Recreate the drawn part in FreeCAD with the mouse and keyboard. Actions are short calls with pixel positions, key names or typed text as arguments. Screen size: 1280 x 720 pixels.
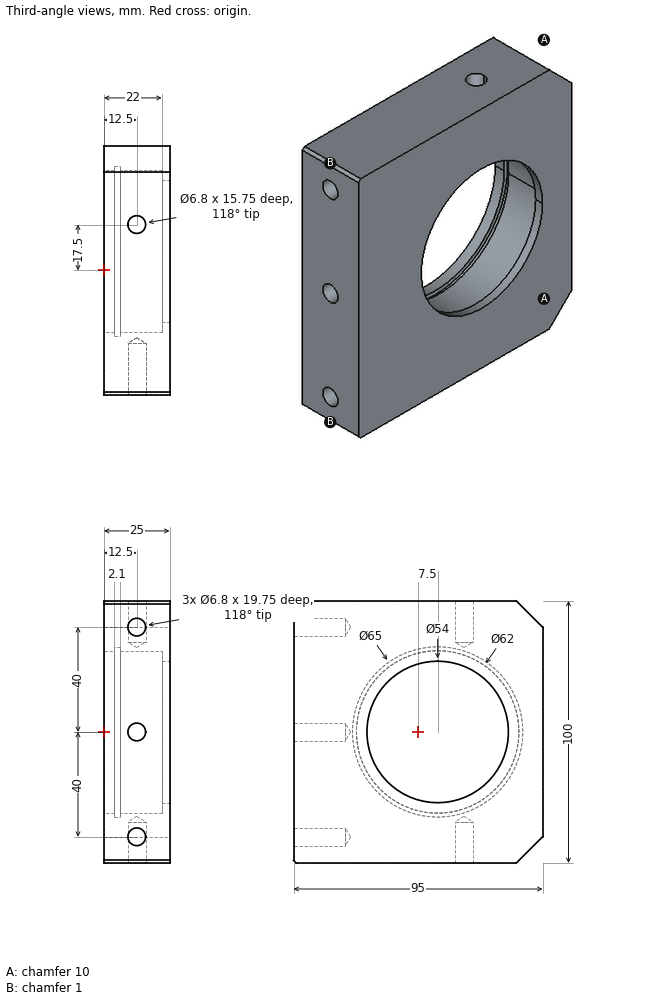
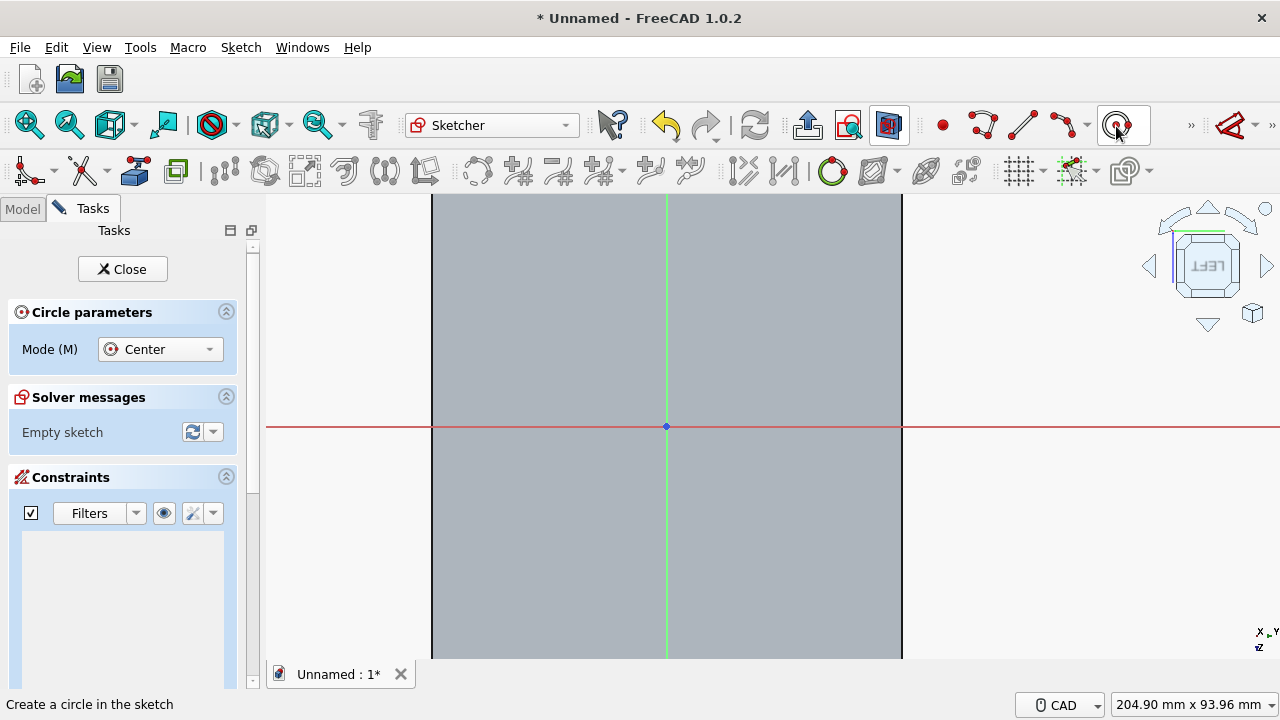
click(704, 426)
click(812, 318)
key(Escape)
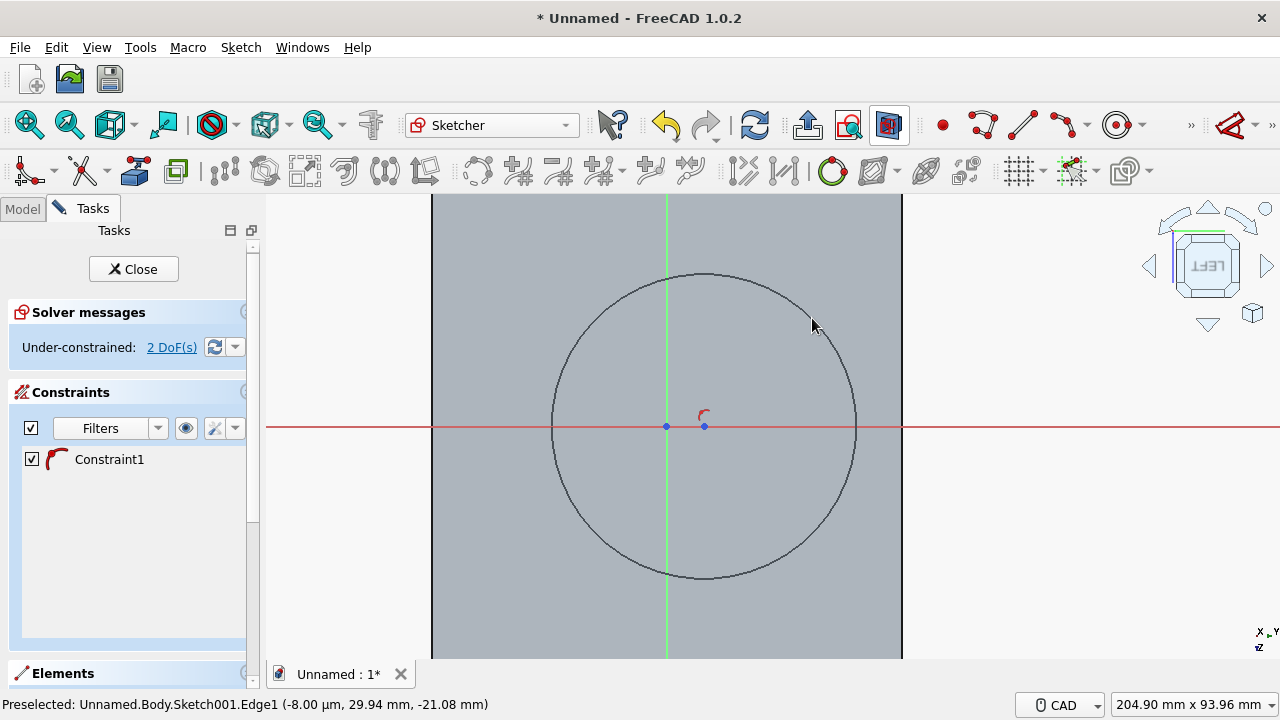
click(1230, 126)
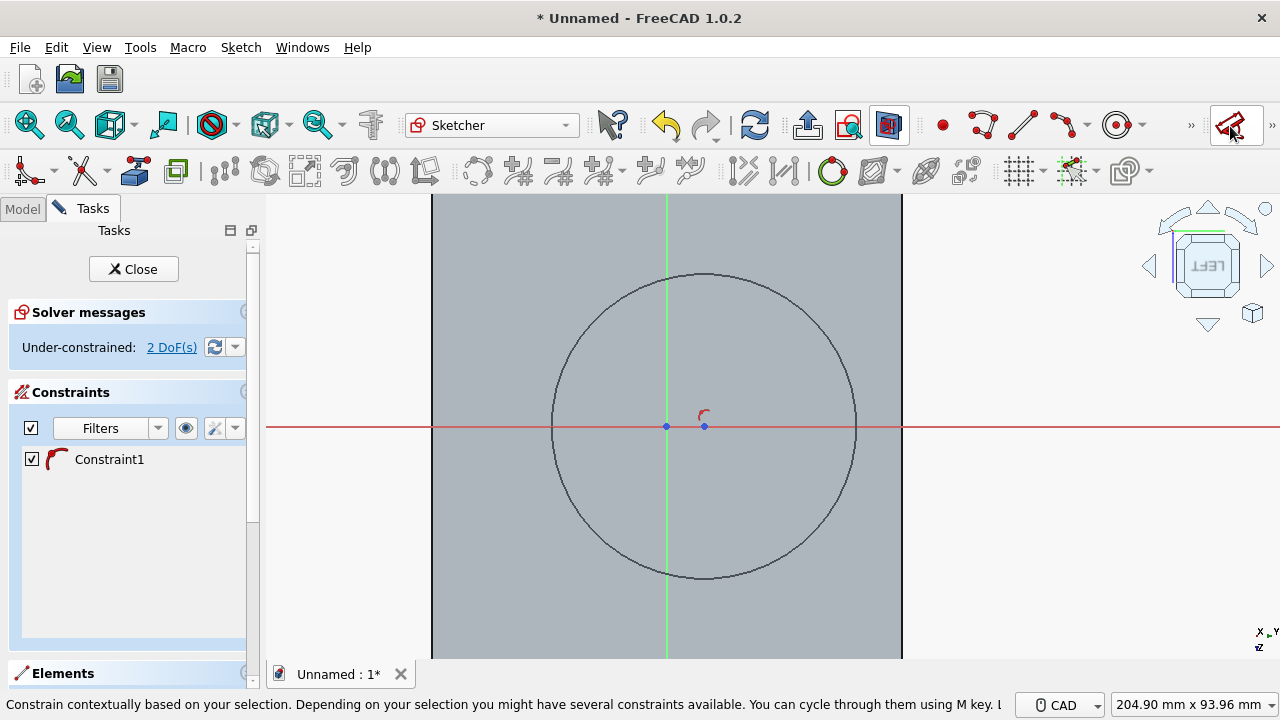
click(811, 318)
click(833, 295)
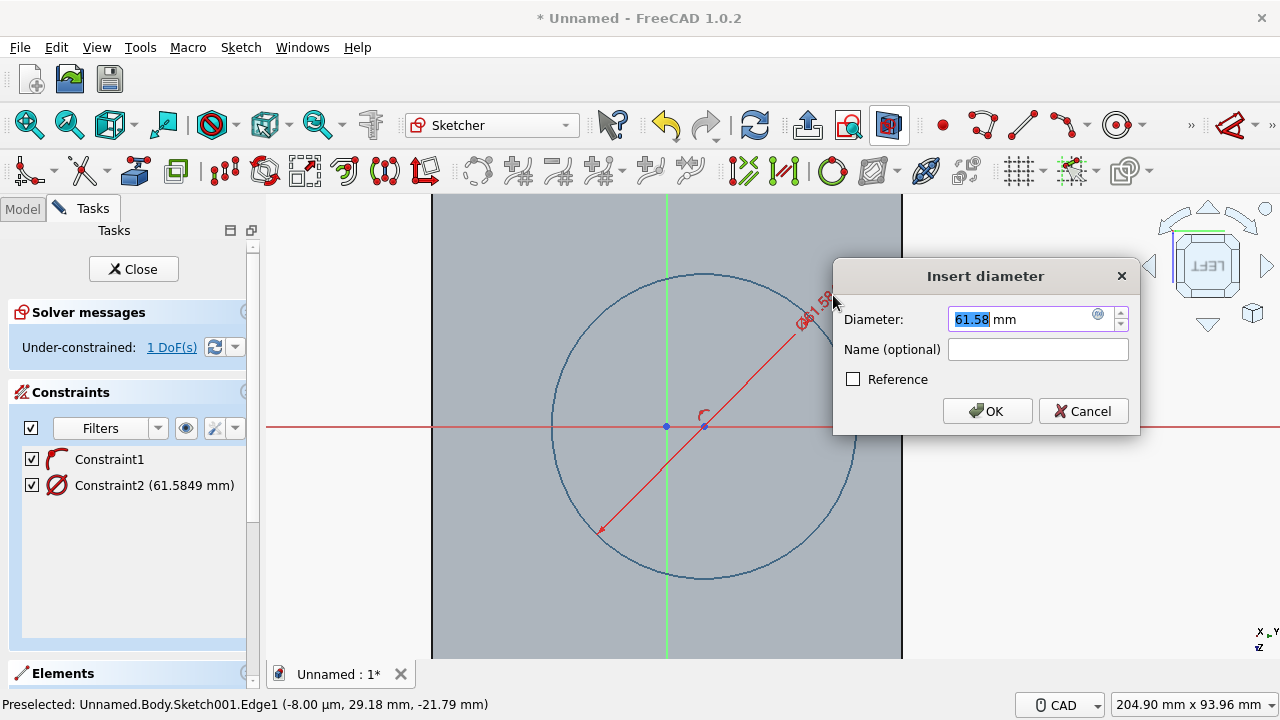
text(62)
key(Return)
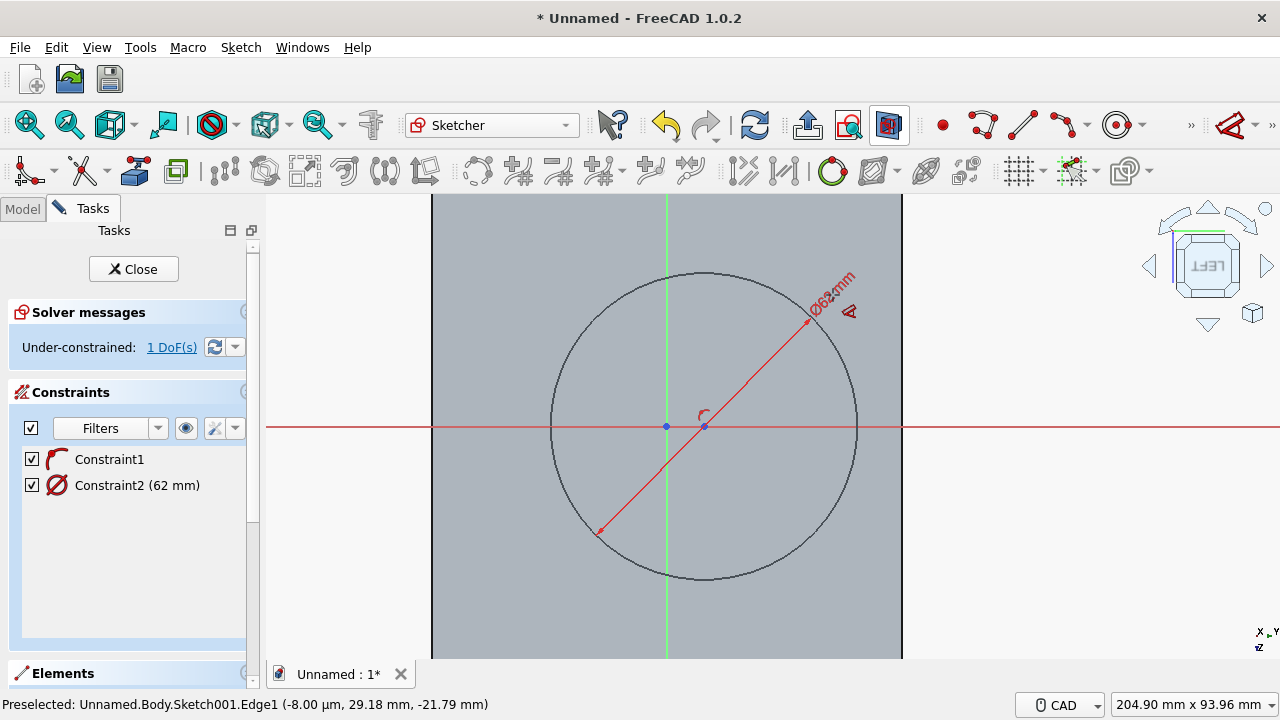
click(704, 426)
click(685, 460)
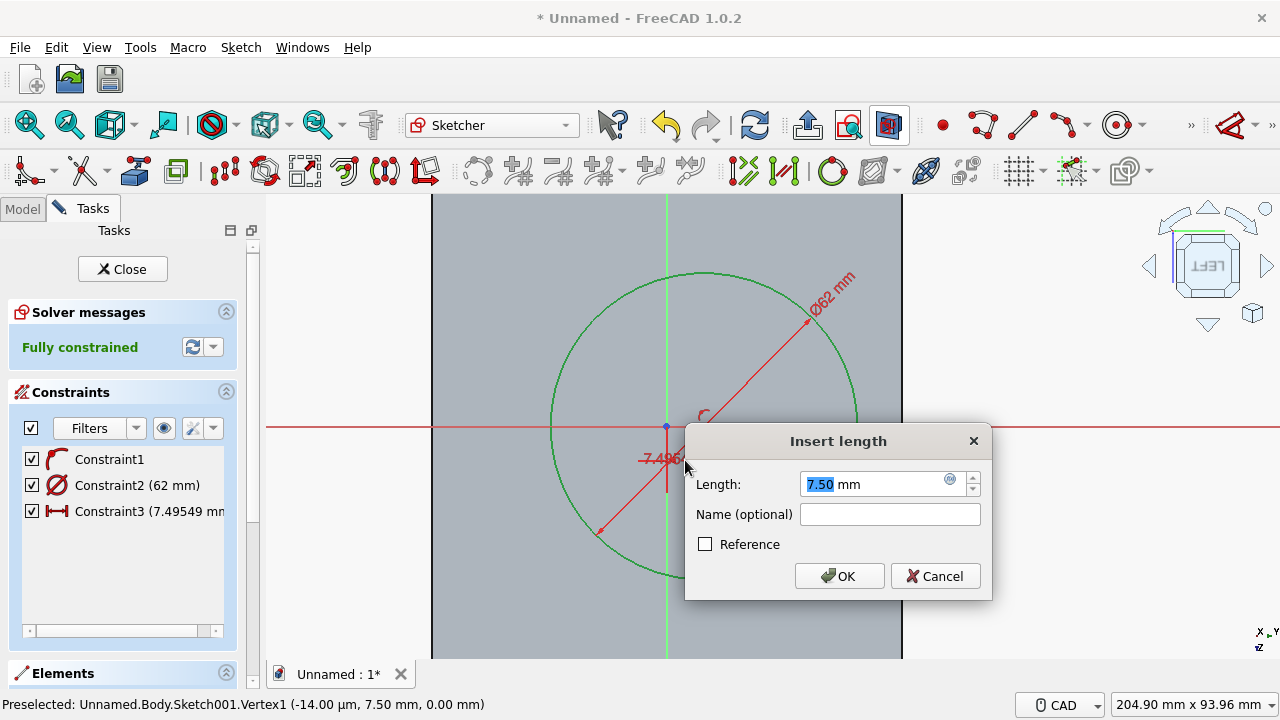
text(7.5)
key(Return)
key(Escape)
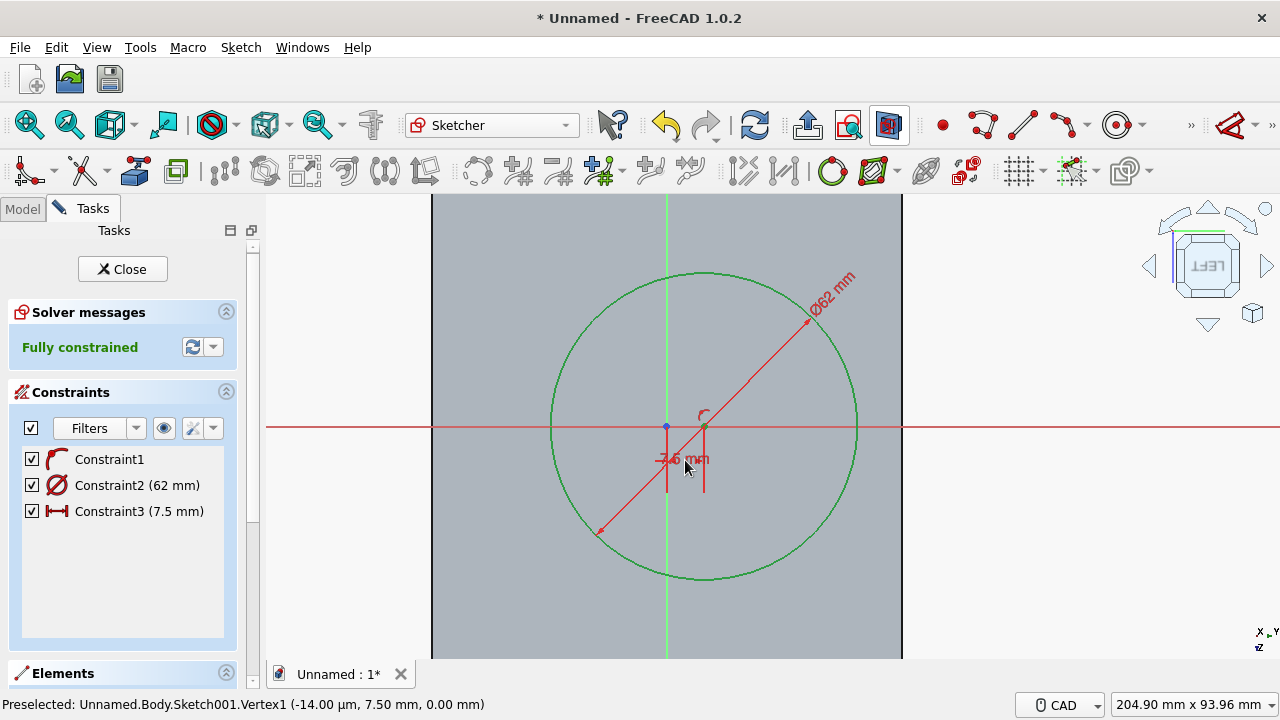
click(123, 269)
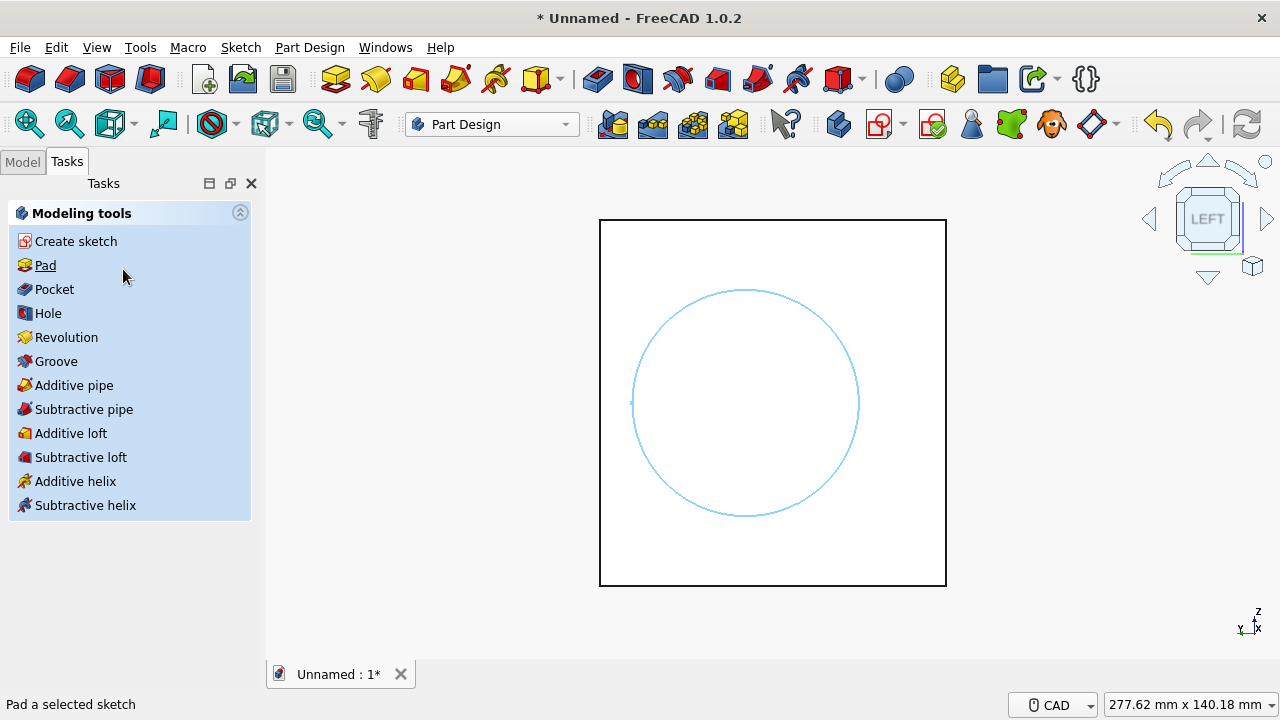
click(598, 80)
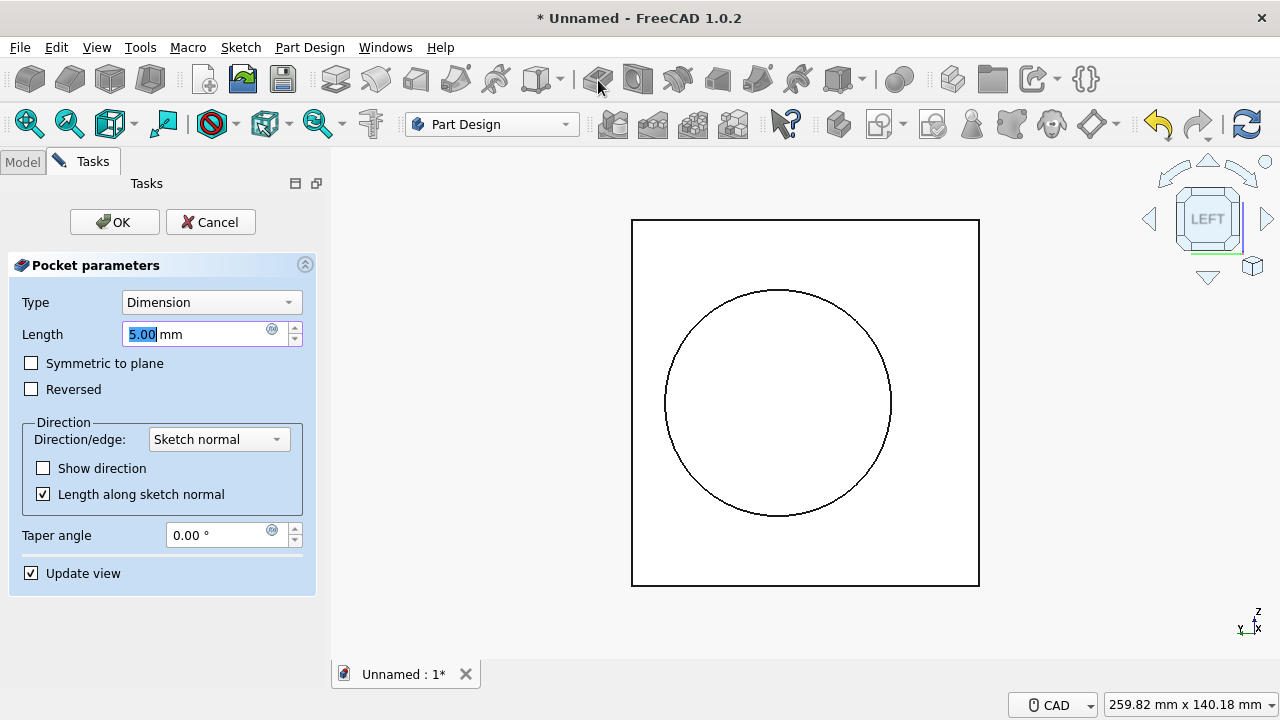
text(22)
key(Tab)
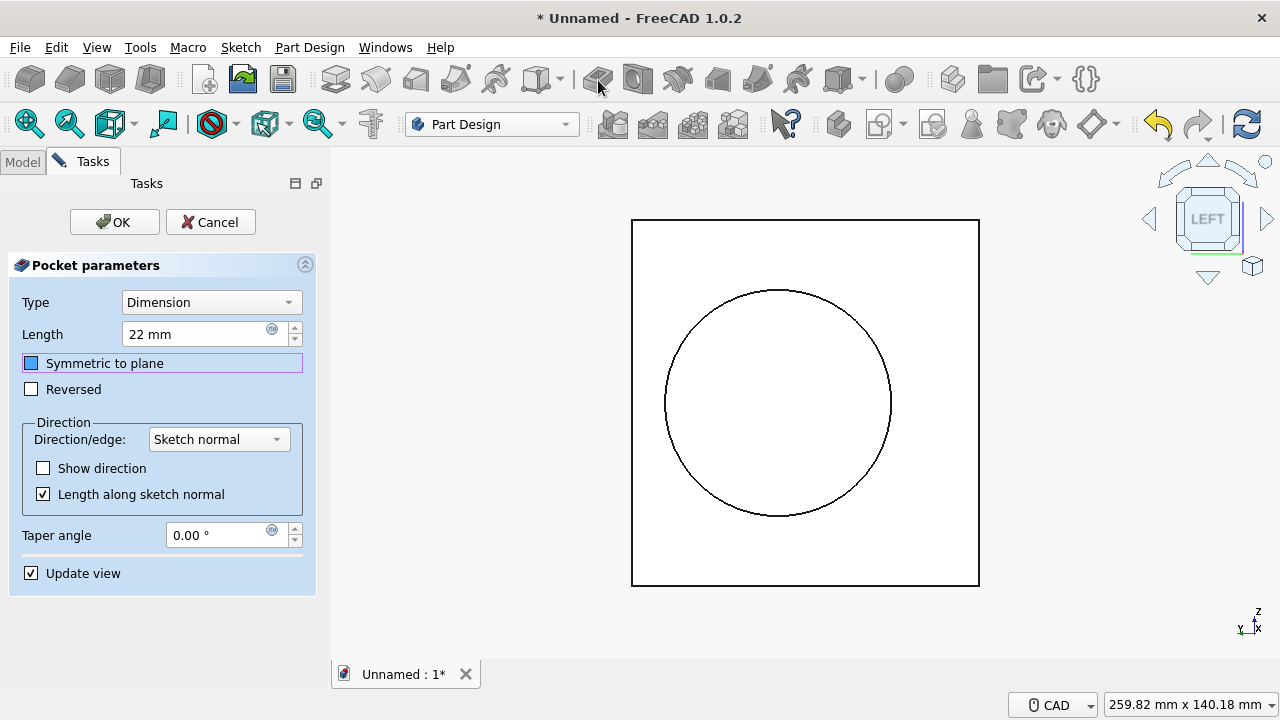
click(115, 222)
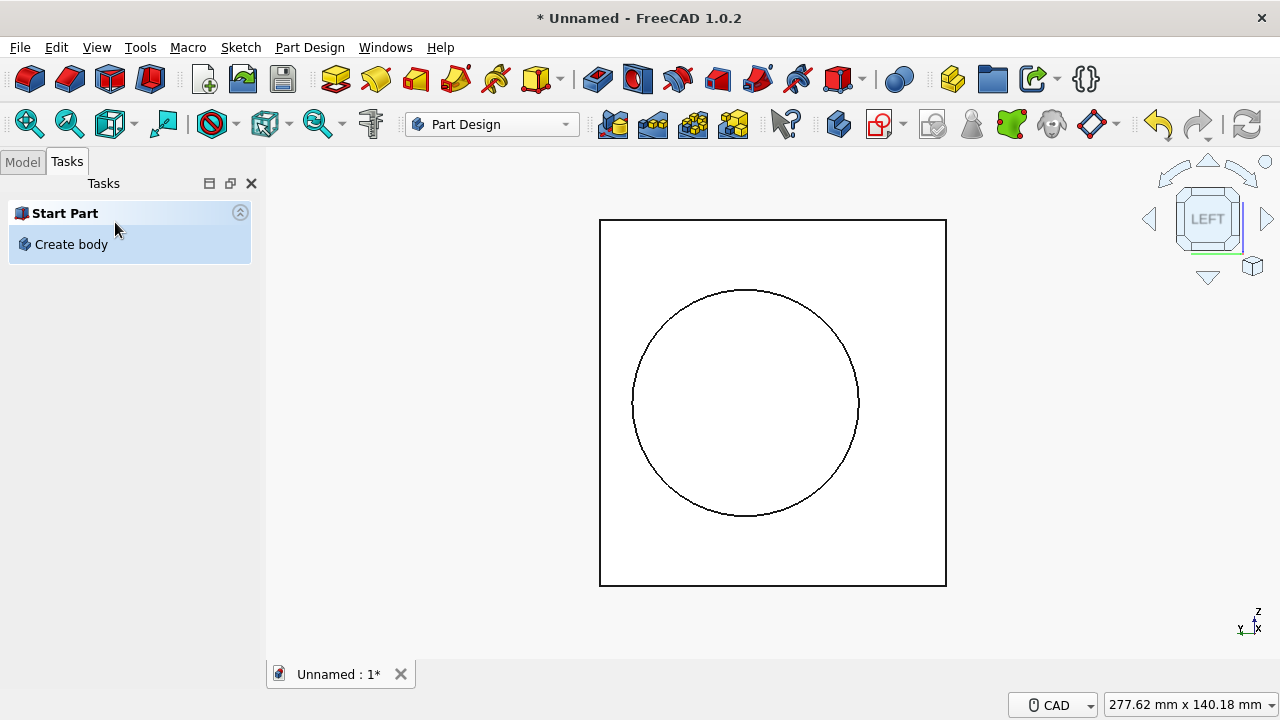
click(746, 402)